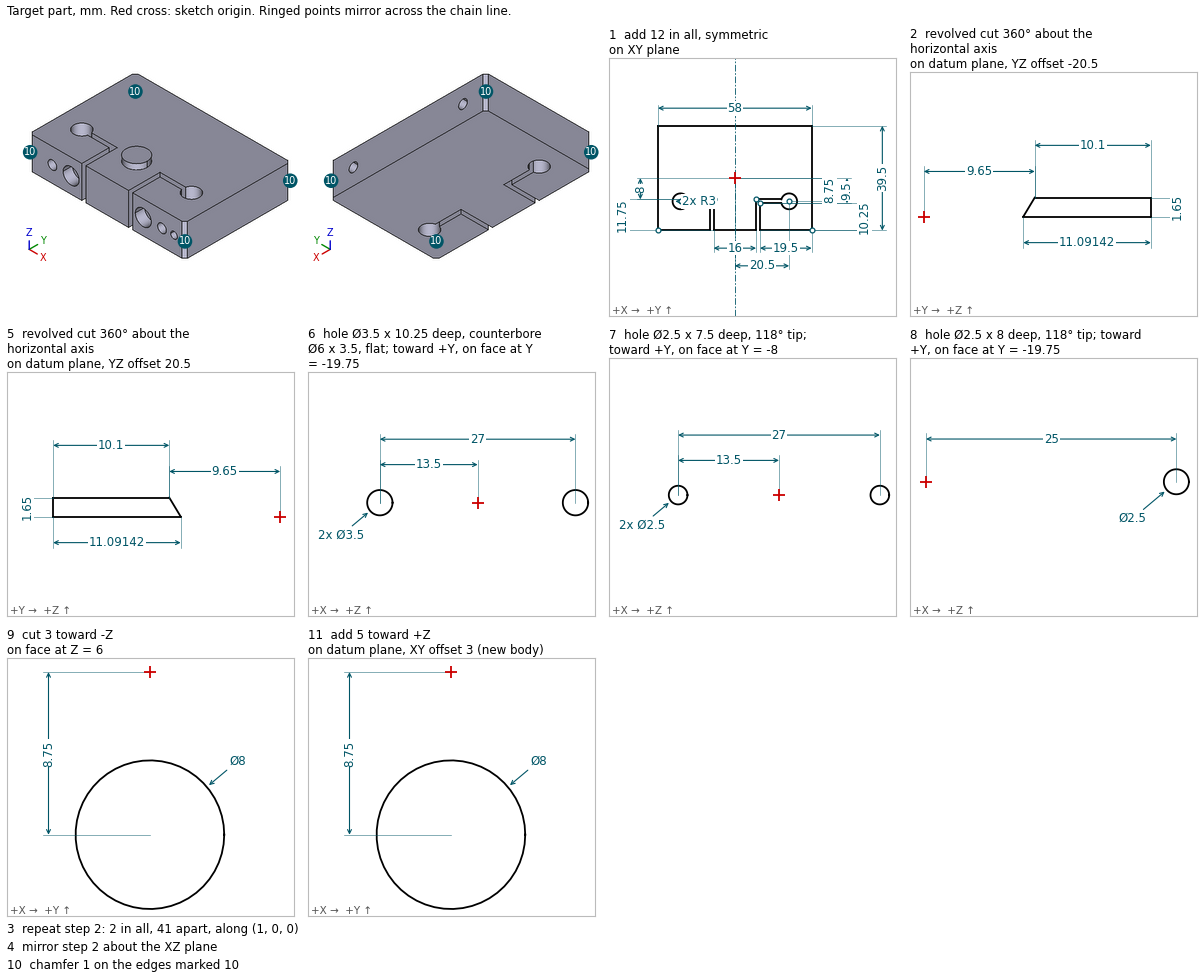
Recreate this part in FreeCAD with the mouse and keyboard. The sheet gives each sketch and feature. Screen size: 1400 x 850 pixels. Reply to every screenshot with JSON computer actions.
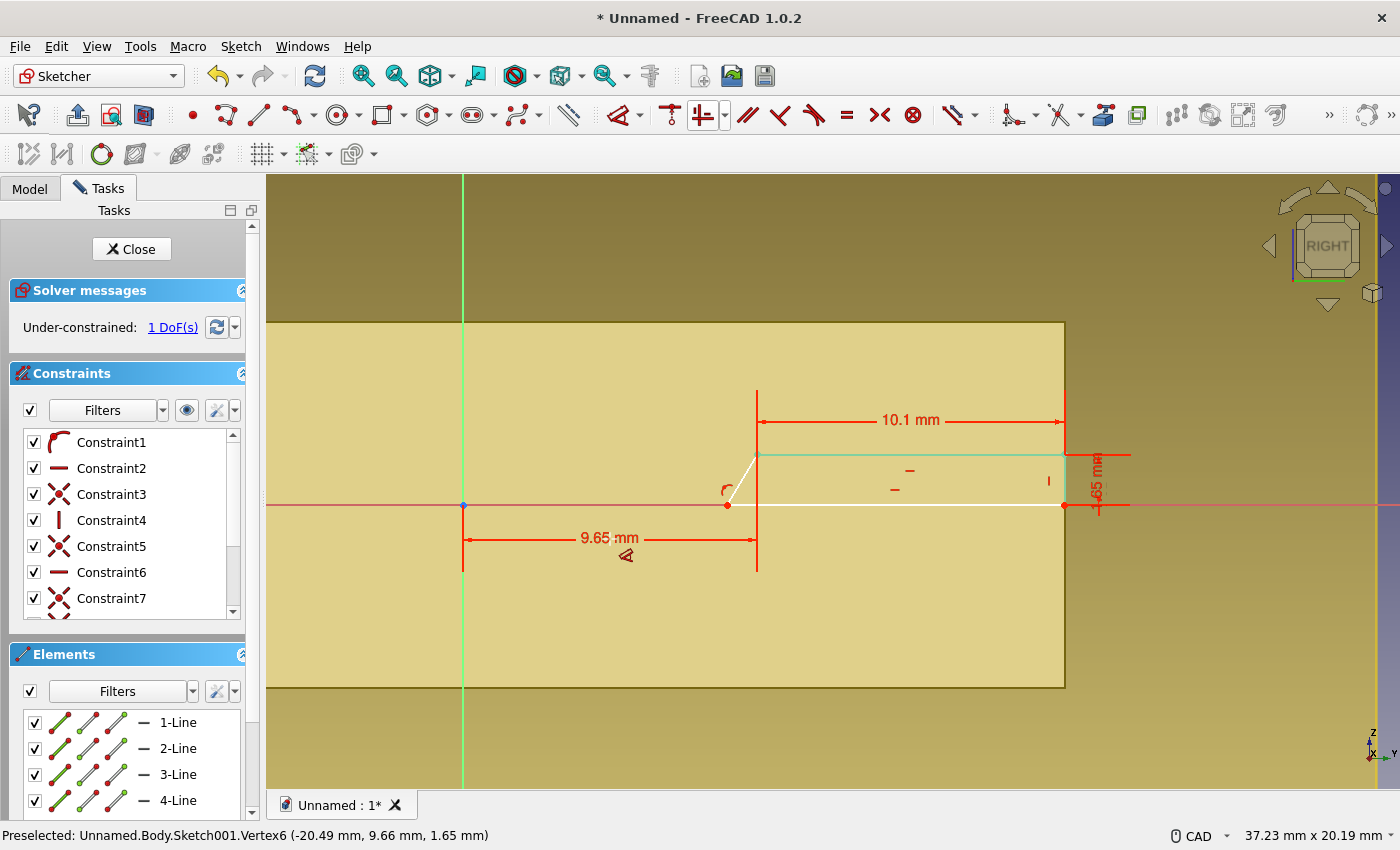
{"action": "left_click", "coordinate": [828, 505]}
{"action": "left_click", "coordinate": [896, 539]}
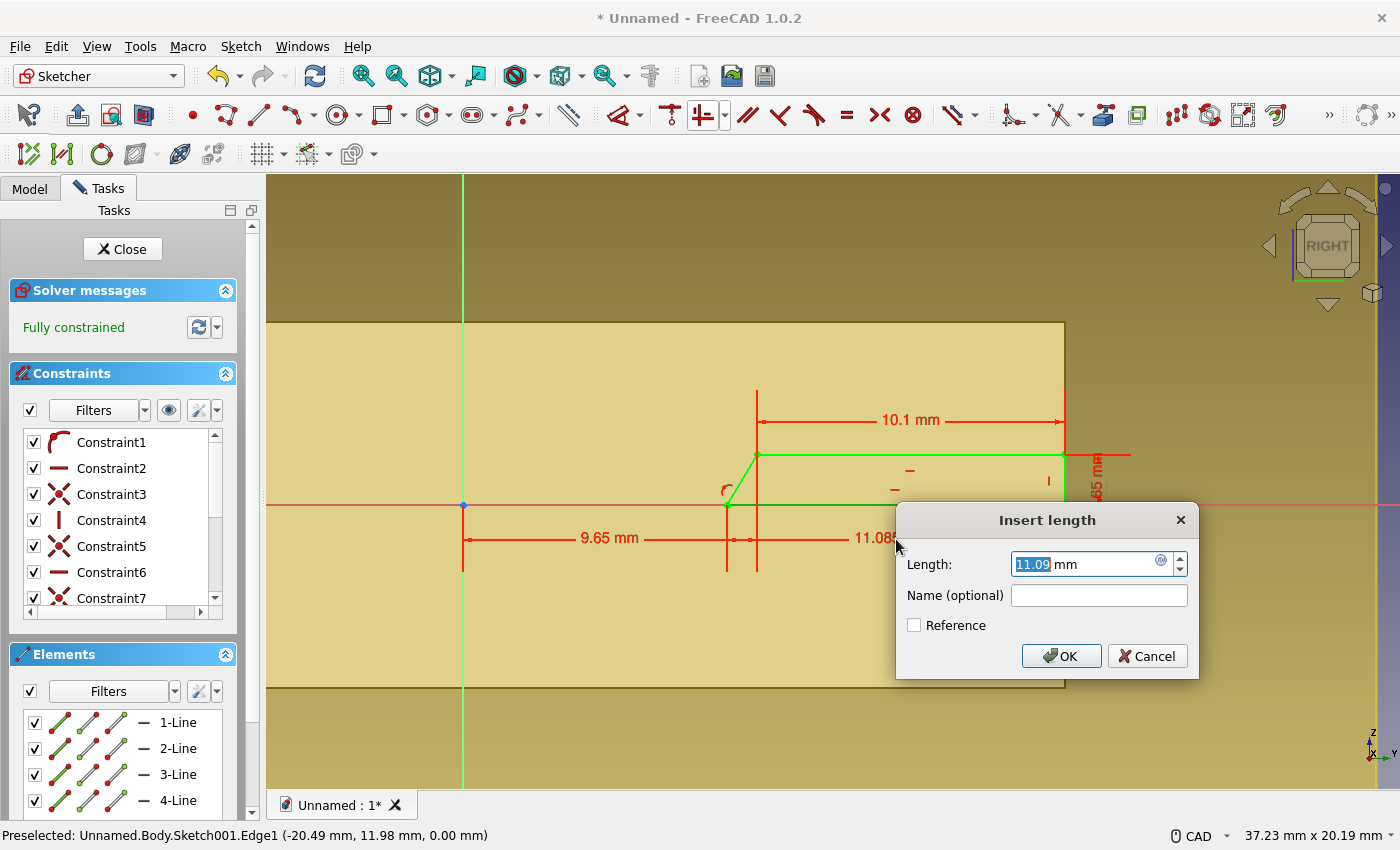
{"action": "type", "text": "11.09142"}
{"action": "key", "text": "Return"}
{"action": "key", "text": "Escape"}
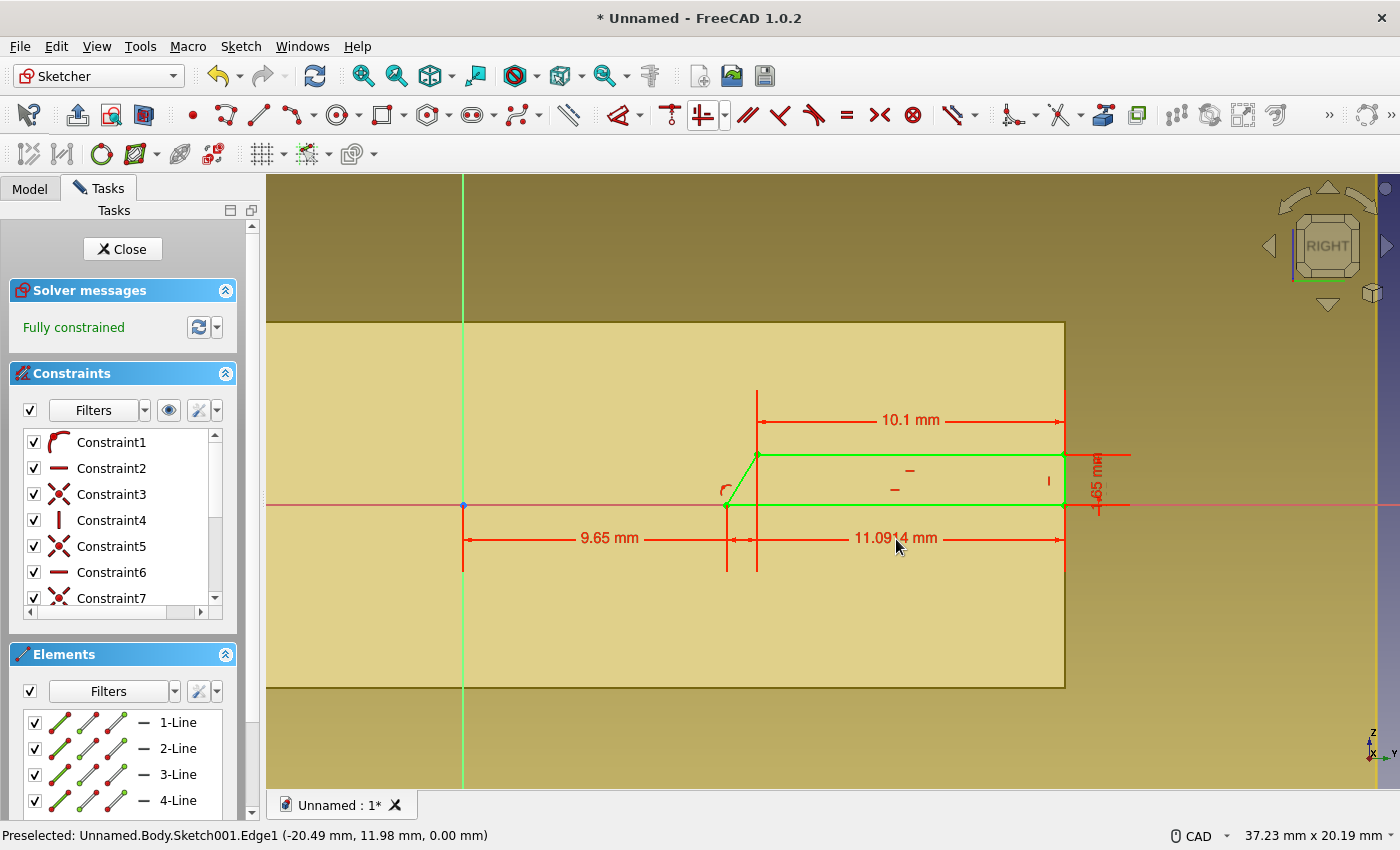
{"action": "left_click", "coordinate": [123, 249]}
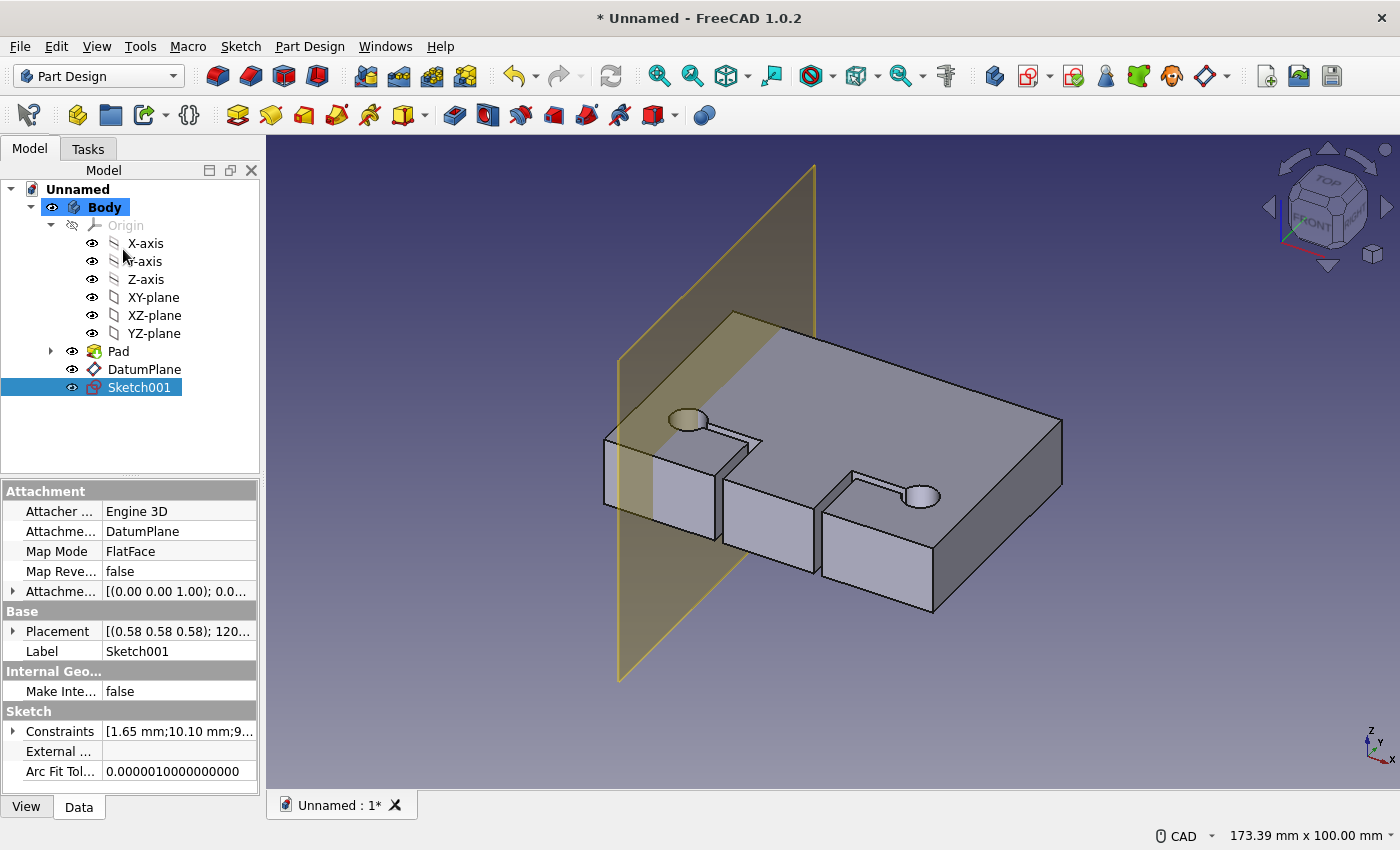
{"action": "left_click", "coordinate": [521, 116]}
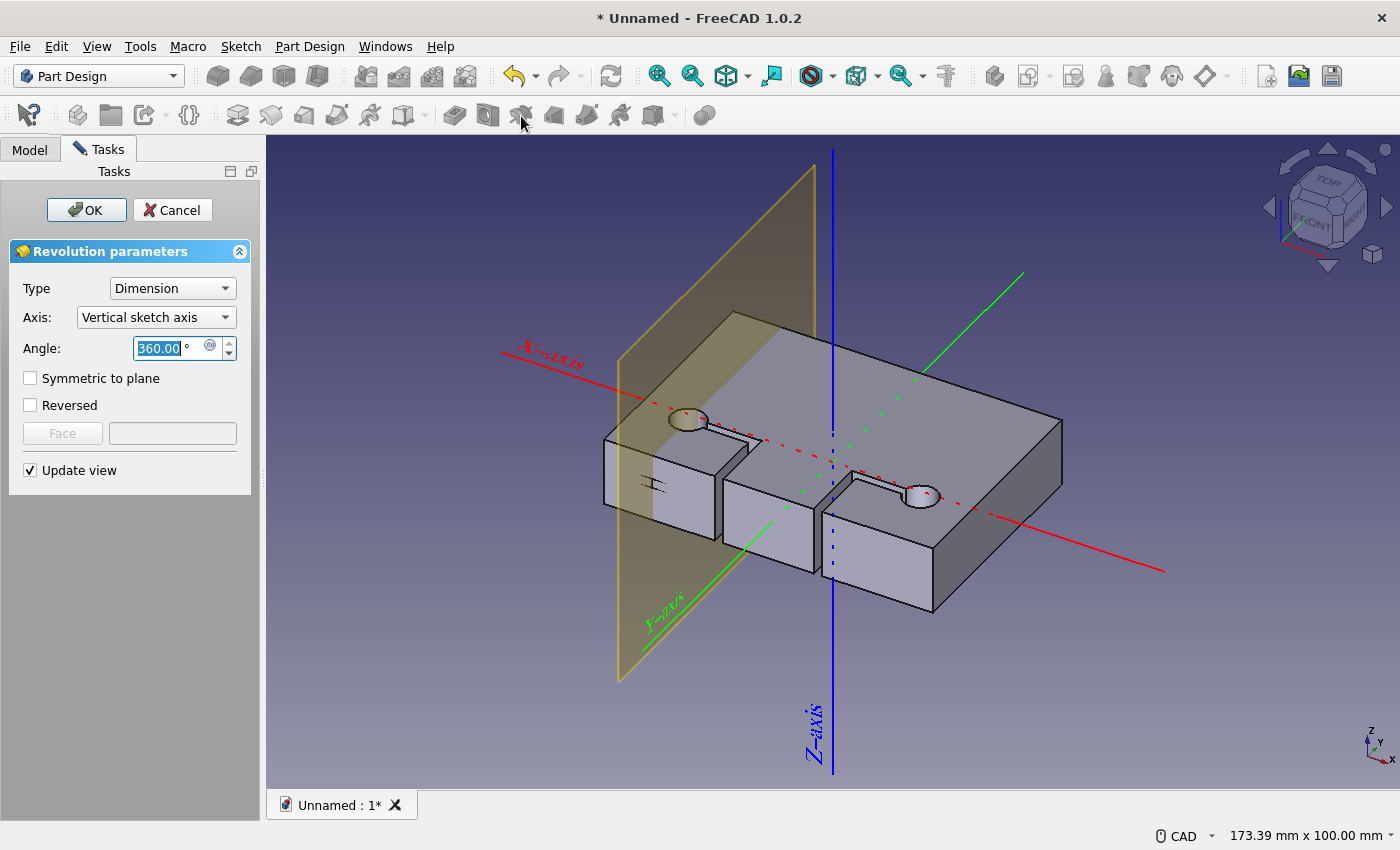
{"action": "left_click", "coordinate": [157, 318]}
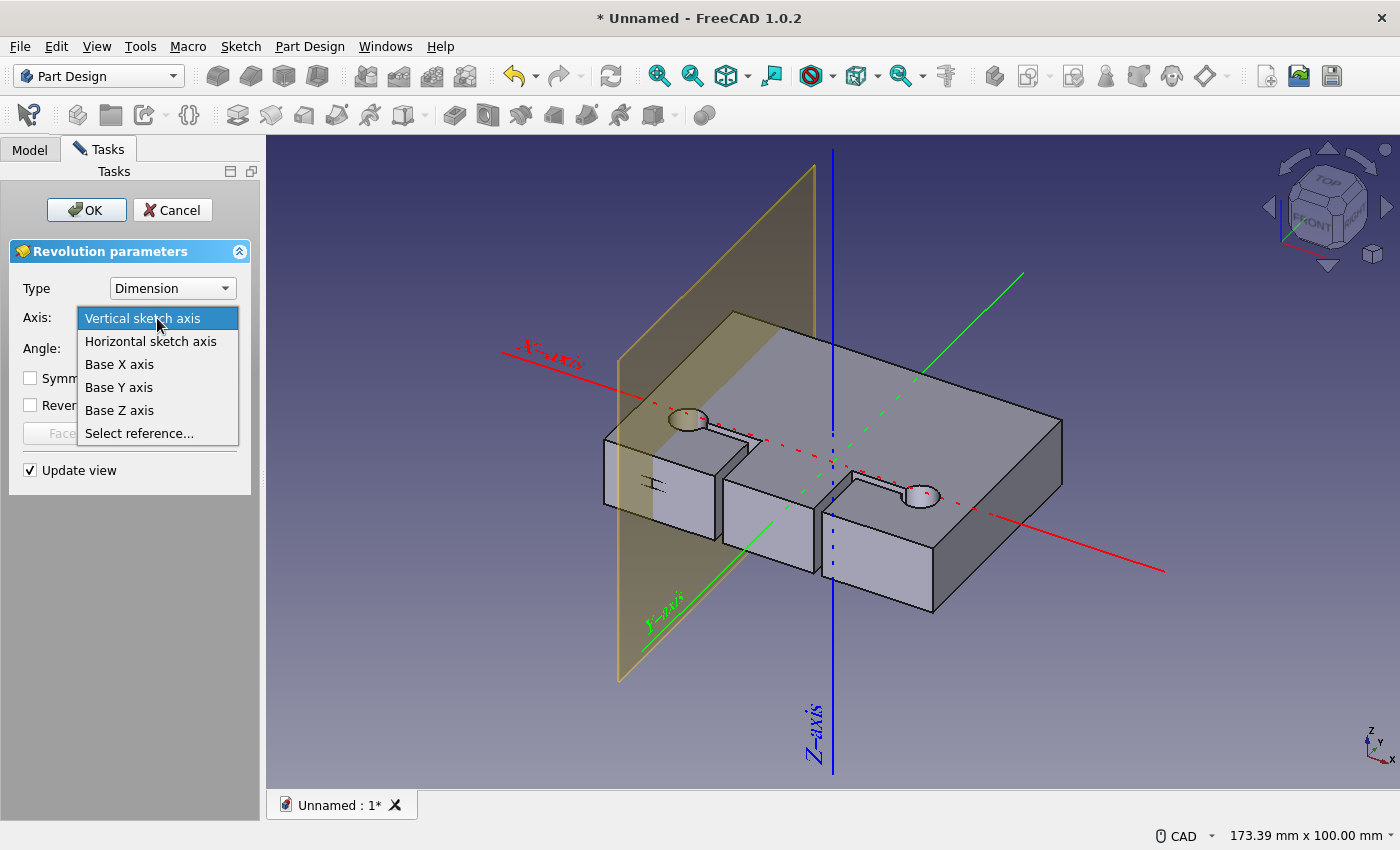
{"action": "left_click", "coordinate": [156, 342]}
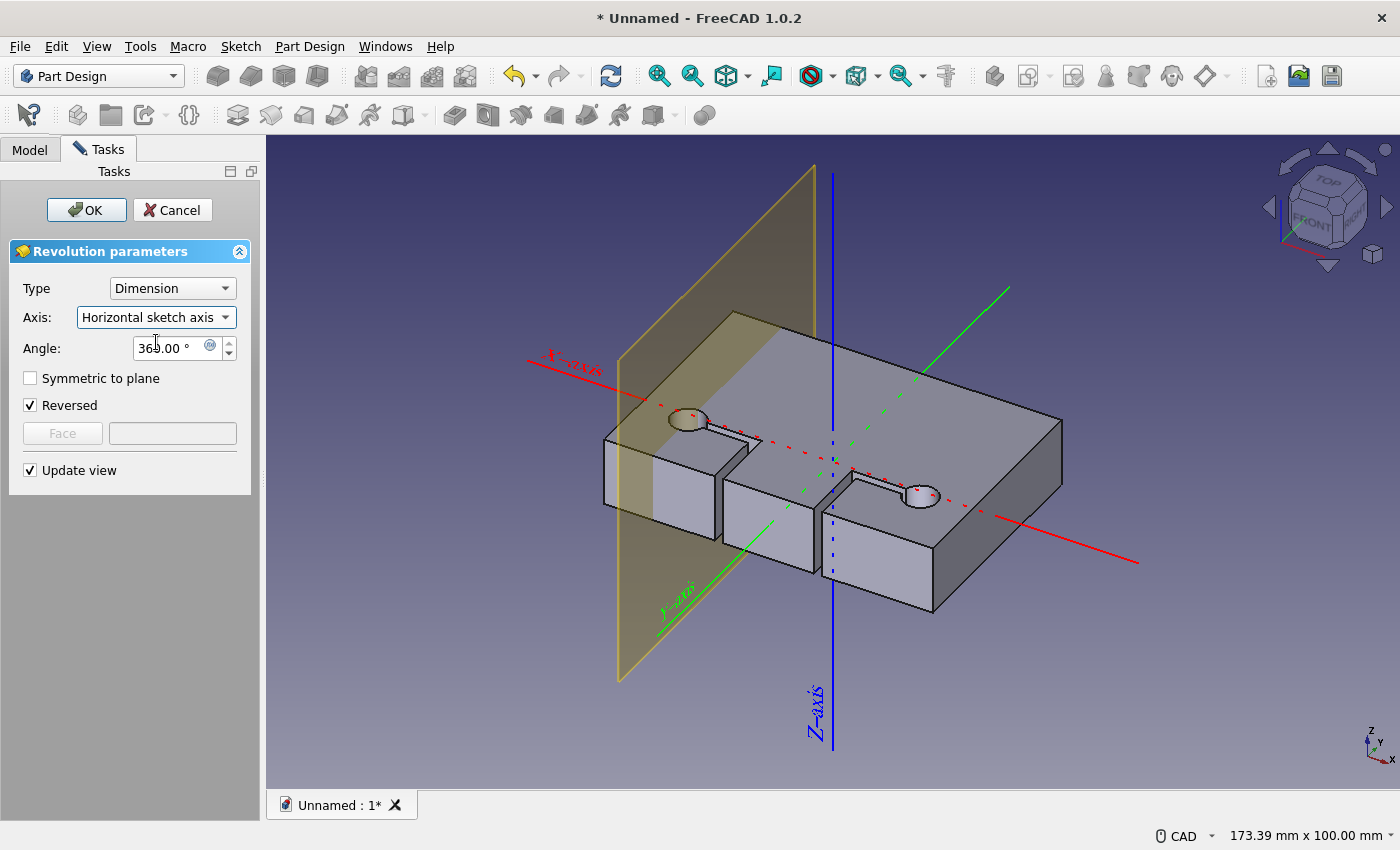
{"action": "left_click", "coordinate": [87, 210]}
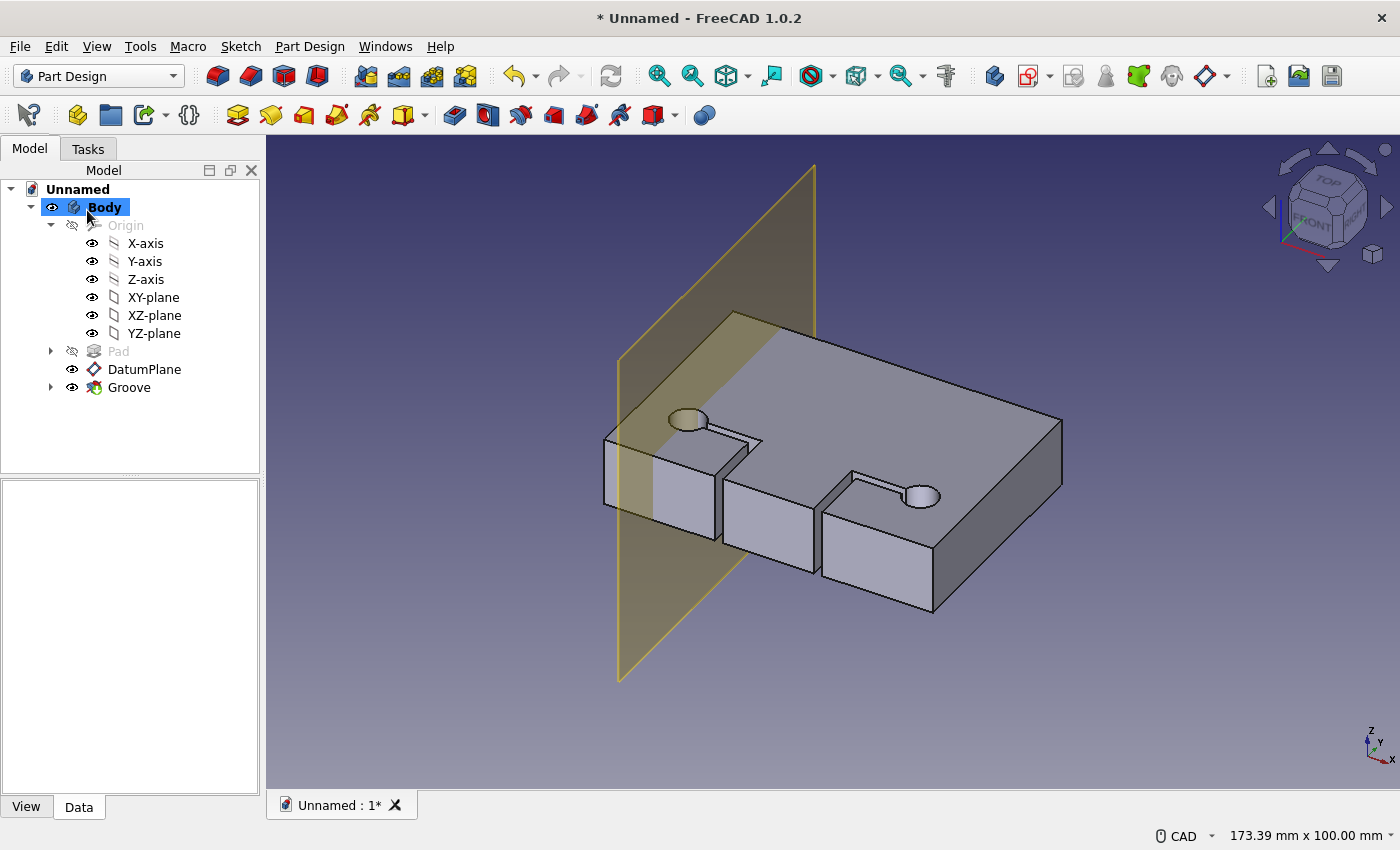
{"action": "left_click", "coordinate": [117, 369]}
{"action": "key", "text": "space"}